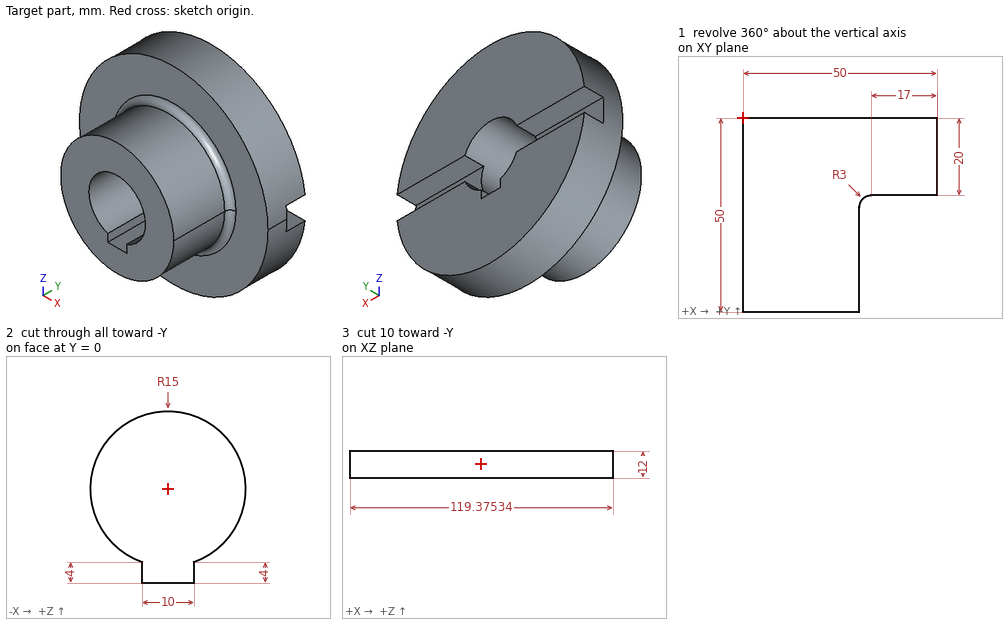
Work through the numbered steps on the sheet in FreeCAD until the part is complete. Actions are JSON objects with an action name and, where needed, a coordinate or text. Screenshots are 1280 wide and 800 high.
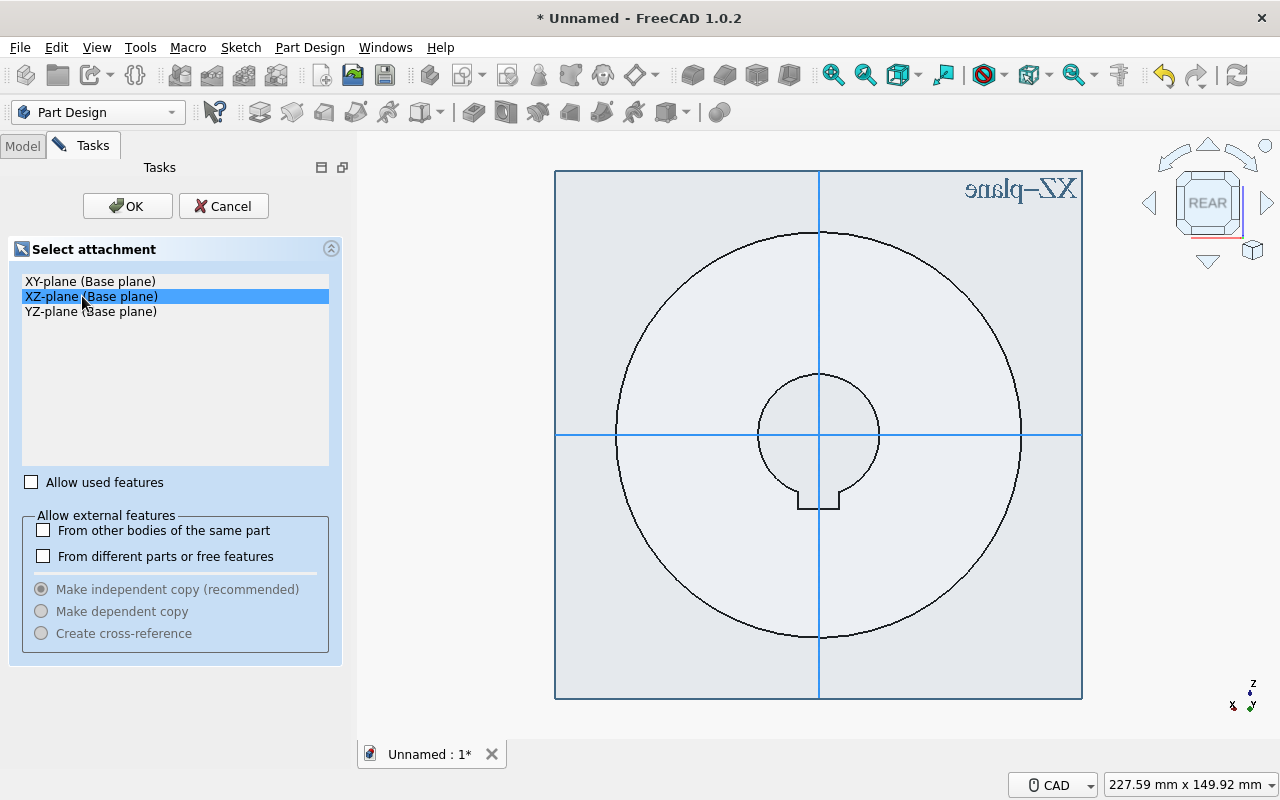
{"action": "left_click", "coordinate": [128, 206]}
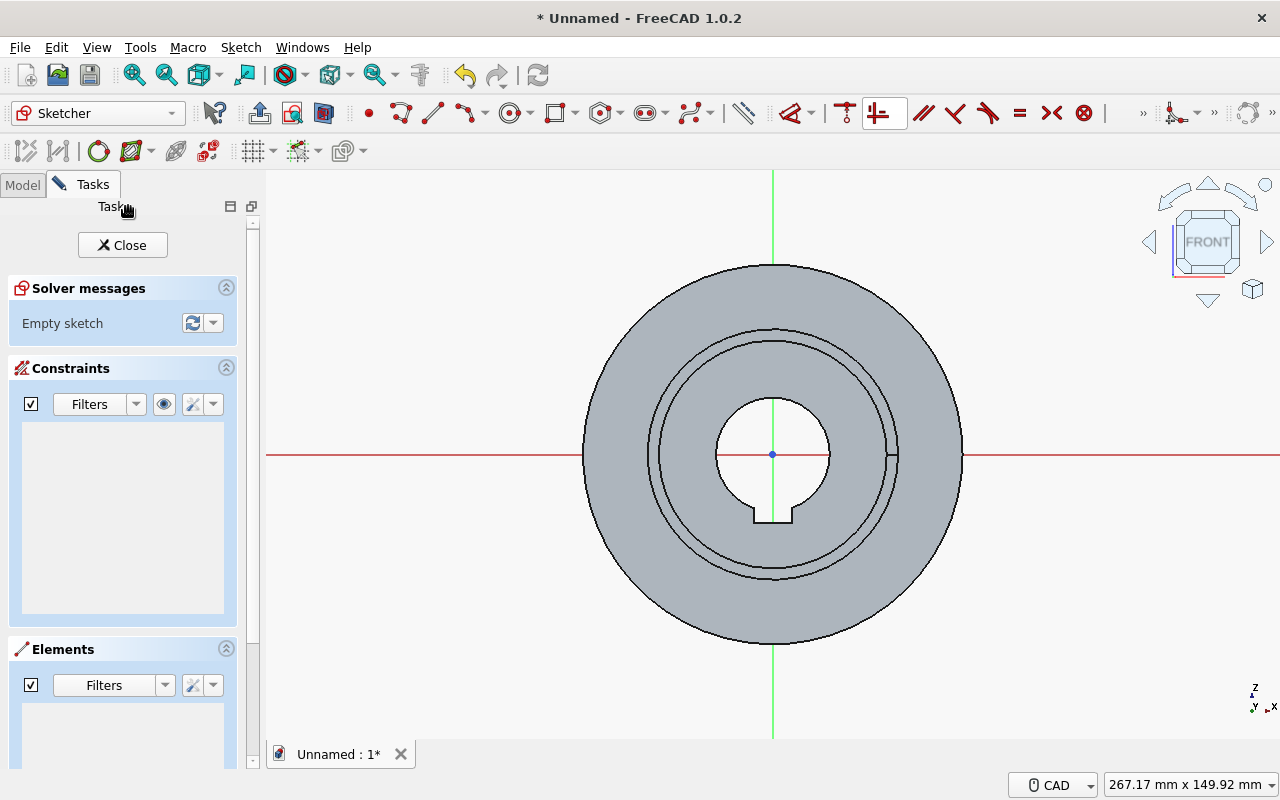
{"action": "left_click", "coordinate": [324, 114]}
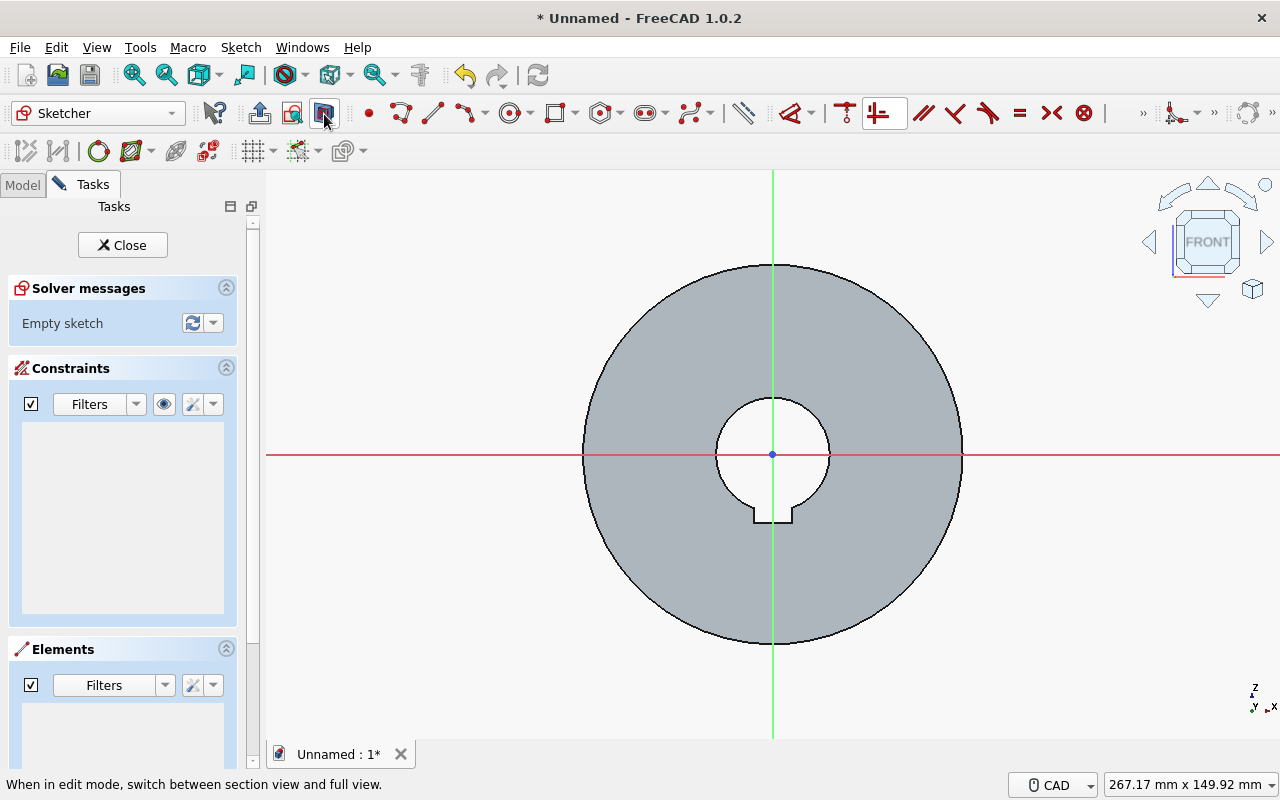
{"action": "key", "text": "g v"}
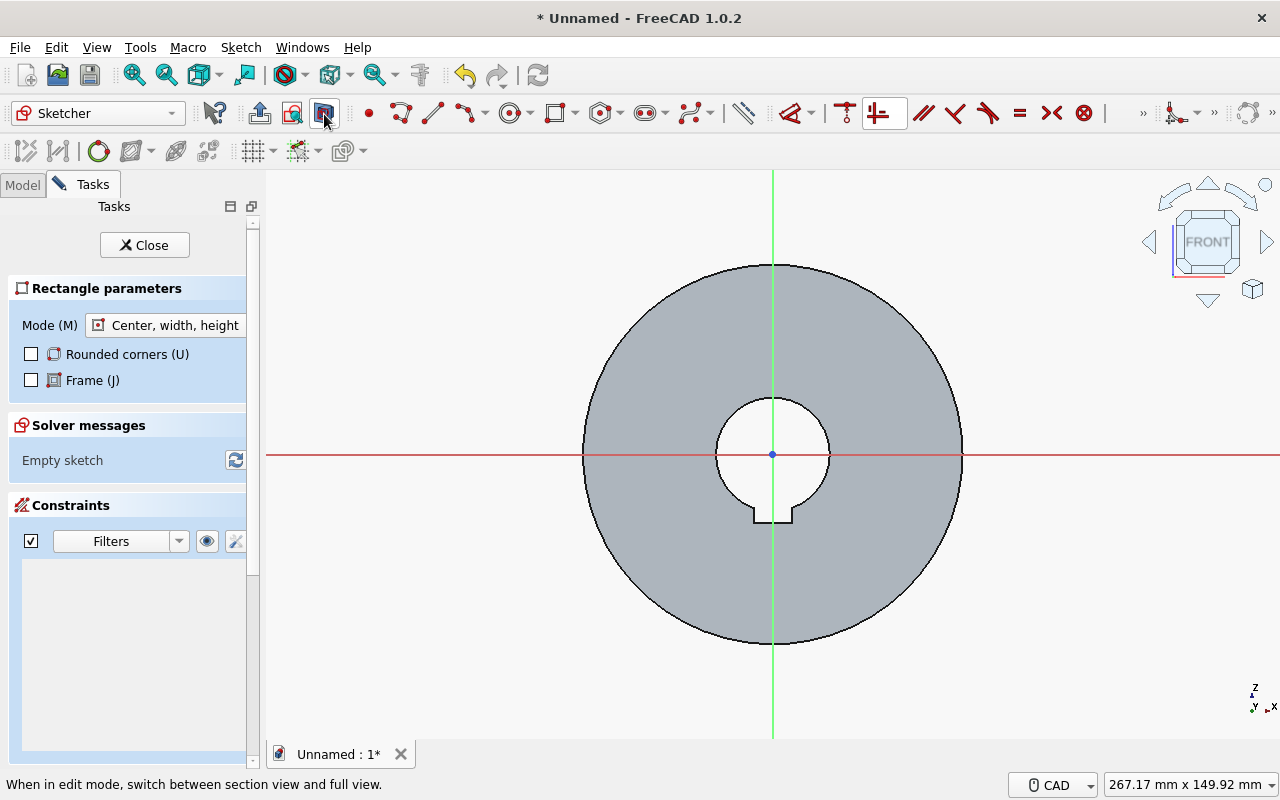
{"action": "left_click", "coordinate": [773, 455]}
{"action": "mouse_move", "coordinate": [999, 432]}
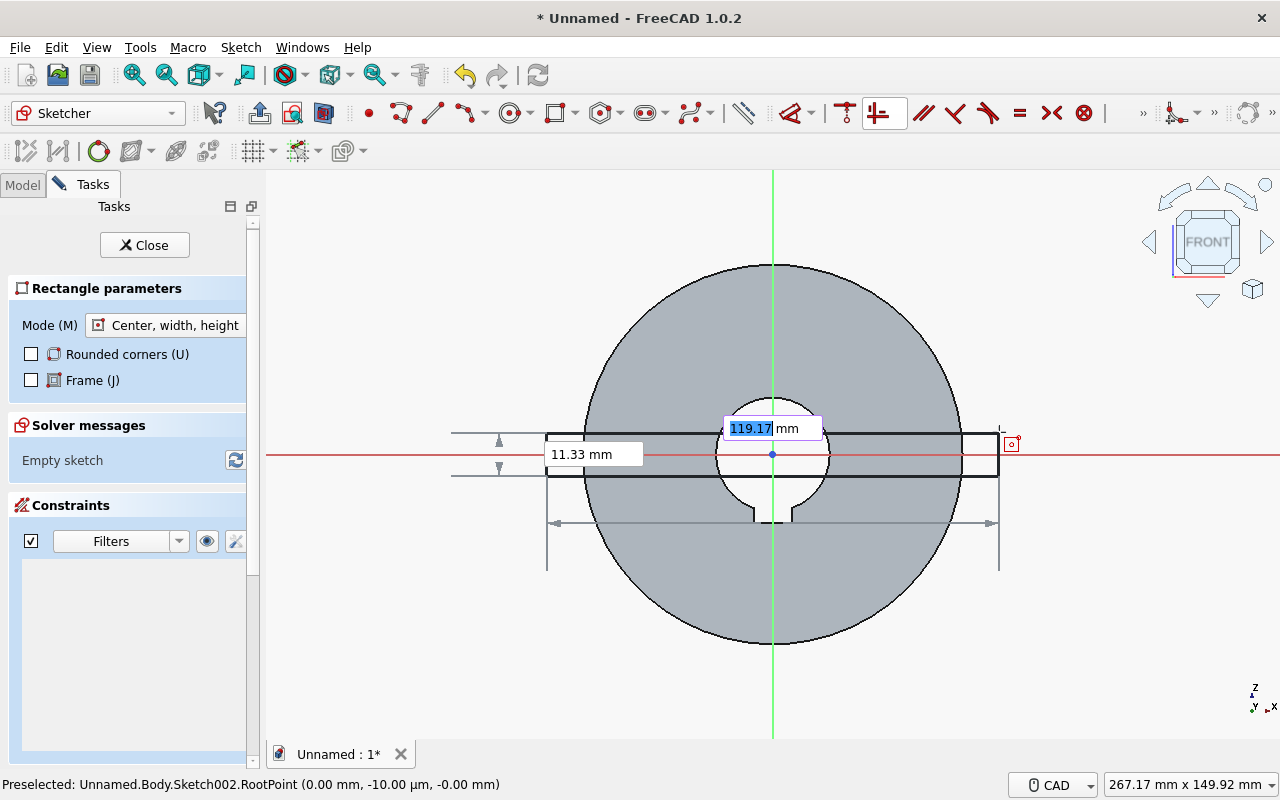
{"action": "type", "text": "119.37534"}
{"action": "key", "text": "Tab"}
{"action": "type", "text": "12"}
{"action": "key", "text": "Return"}
{"action": "key", "text": "Escape"}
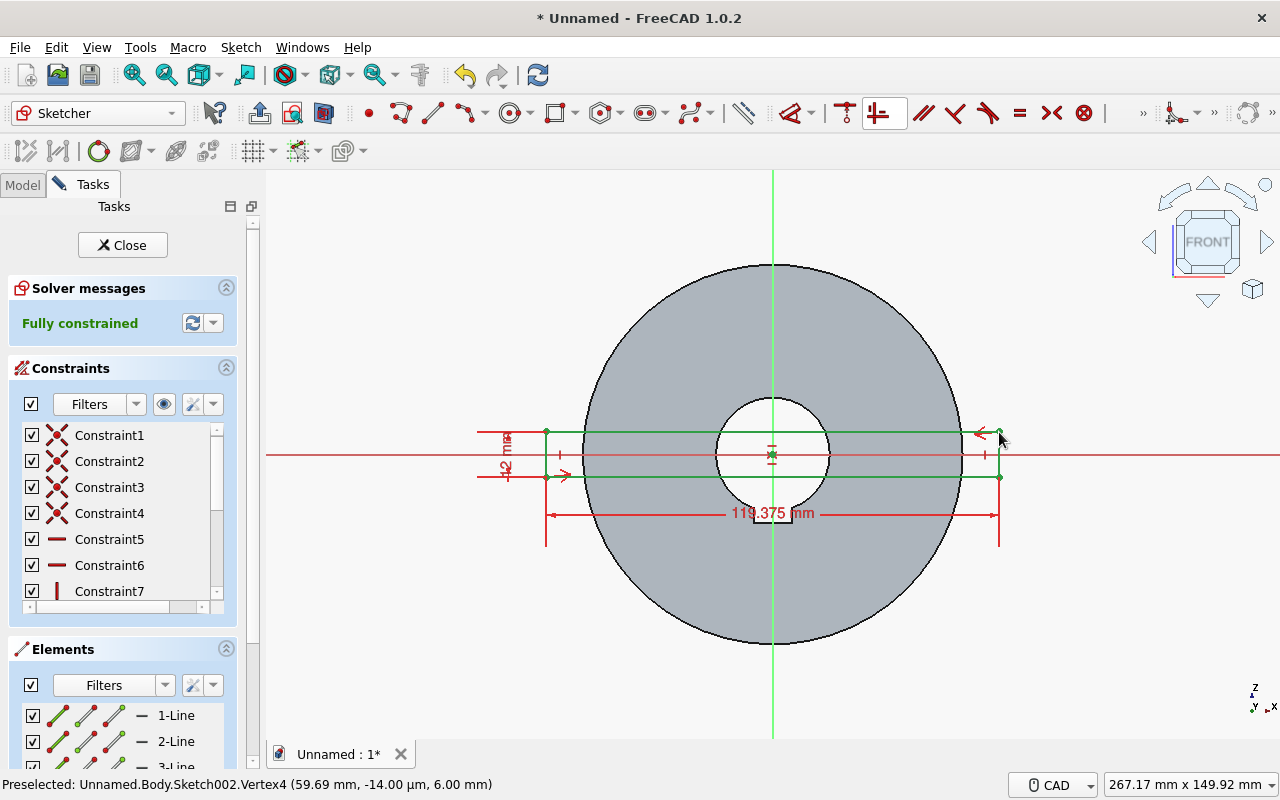
{"action": "left_click", "coordinate": [123, 245]}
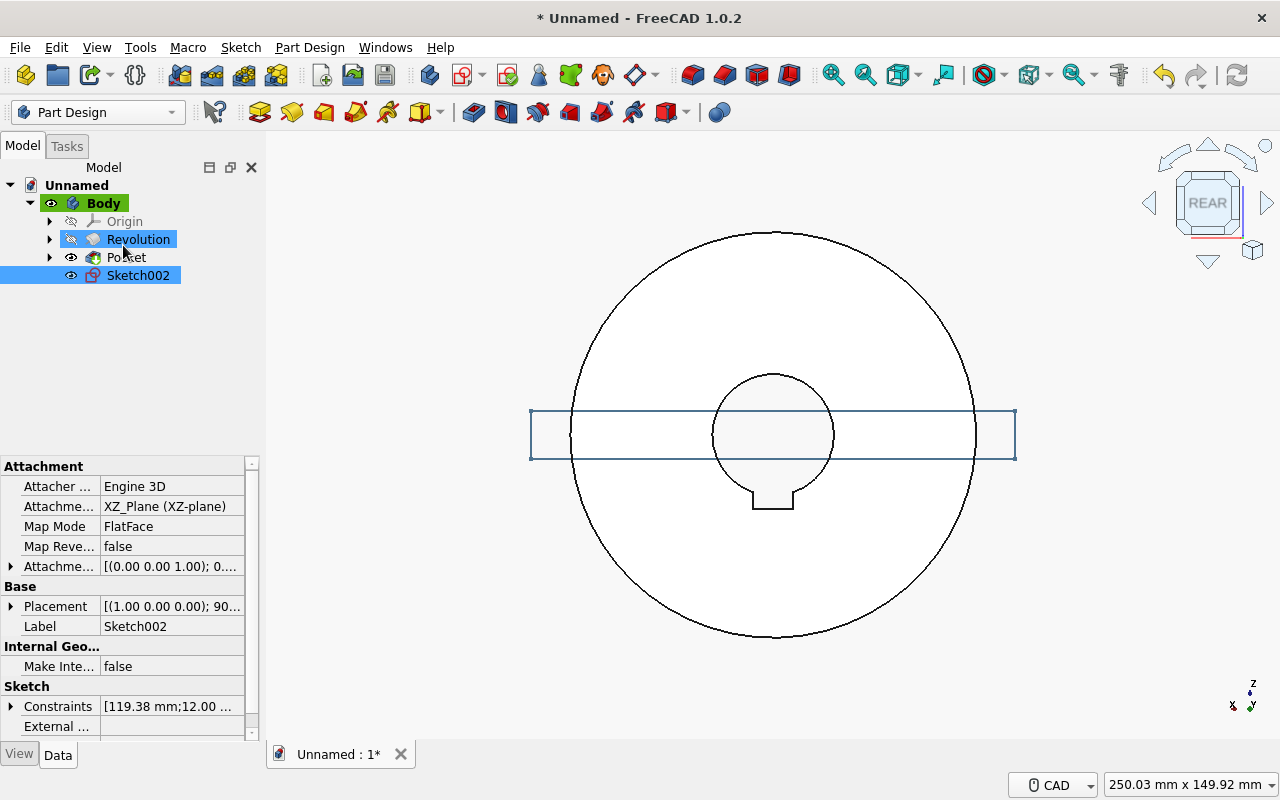
{"action": "left_click", "coordinate": [474, 112]}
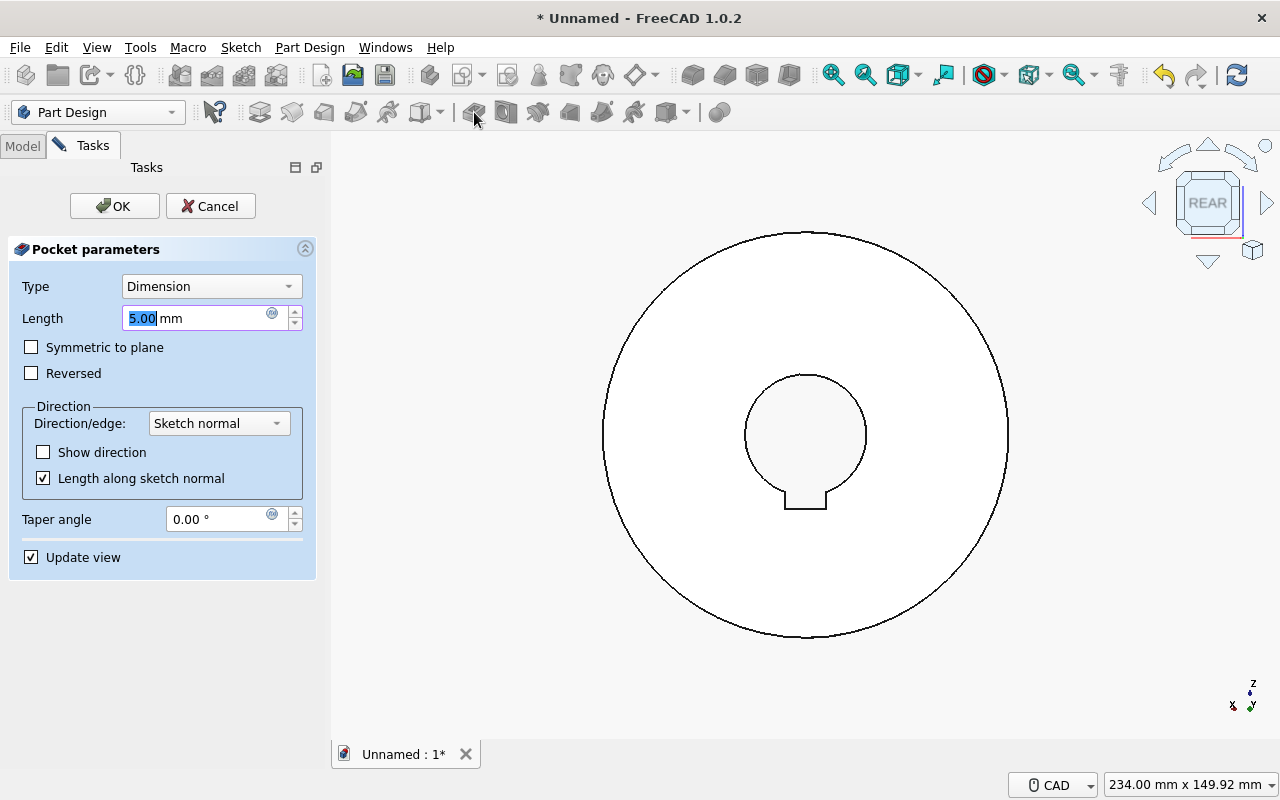
{"action": "type", "text": "10"}
{"action": "key", "text": "Tab"}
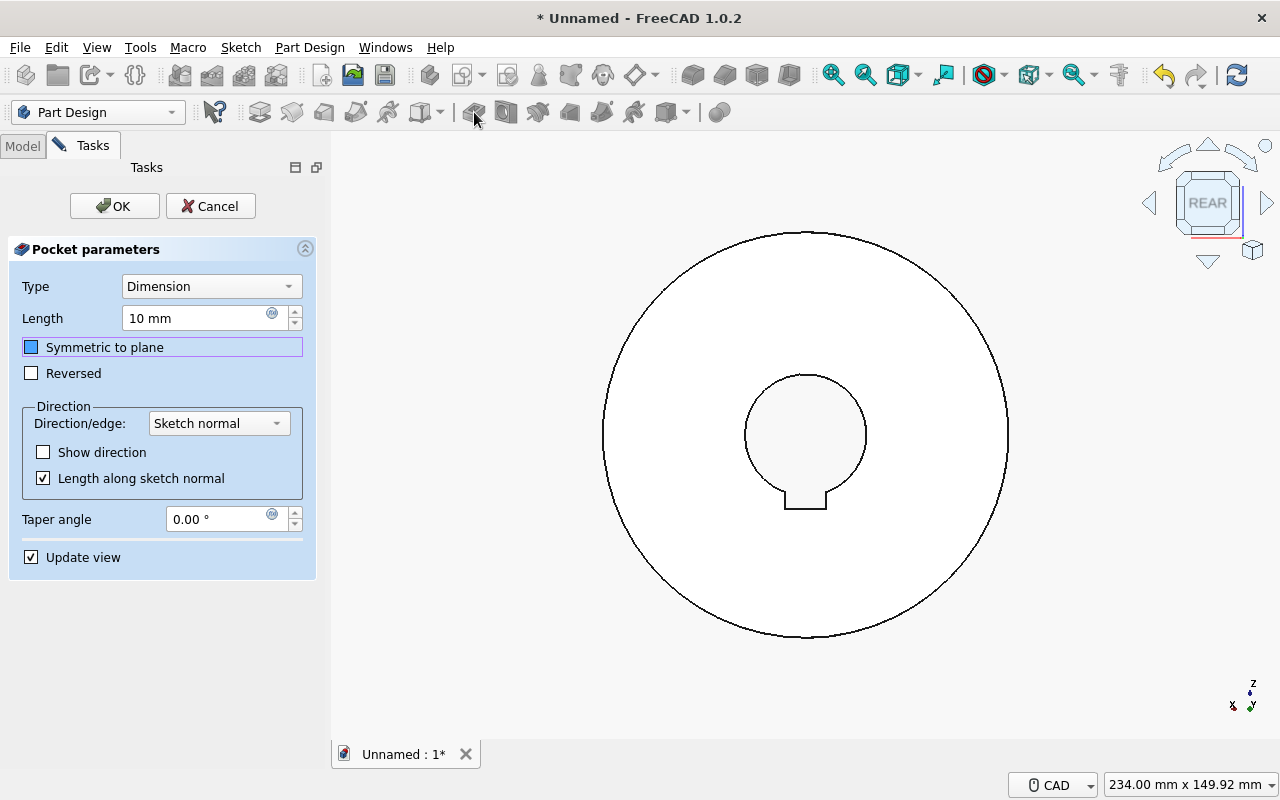
{"action": "left_click", "coordinate": [30, 373]}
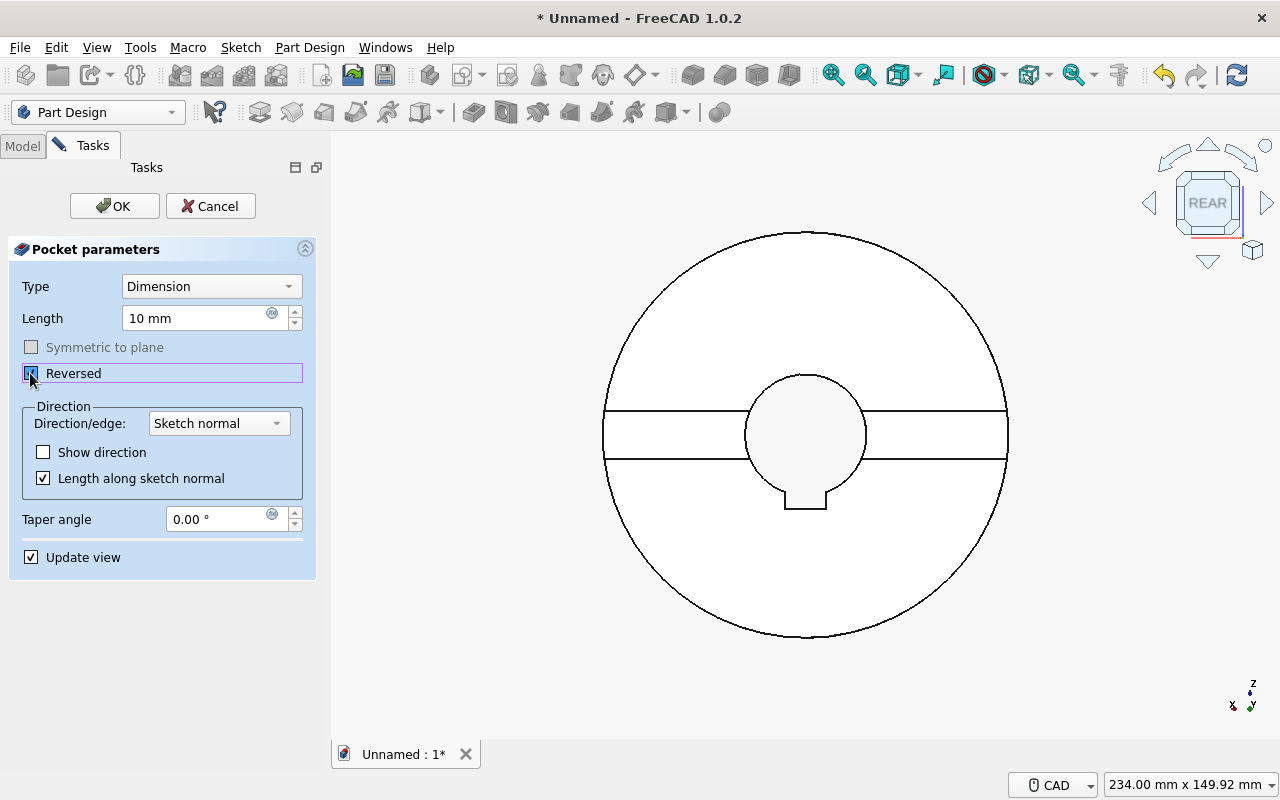
{"action": "left_click", "coordinate": [115, 206]}